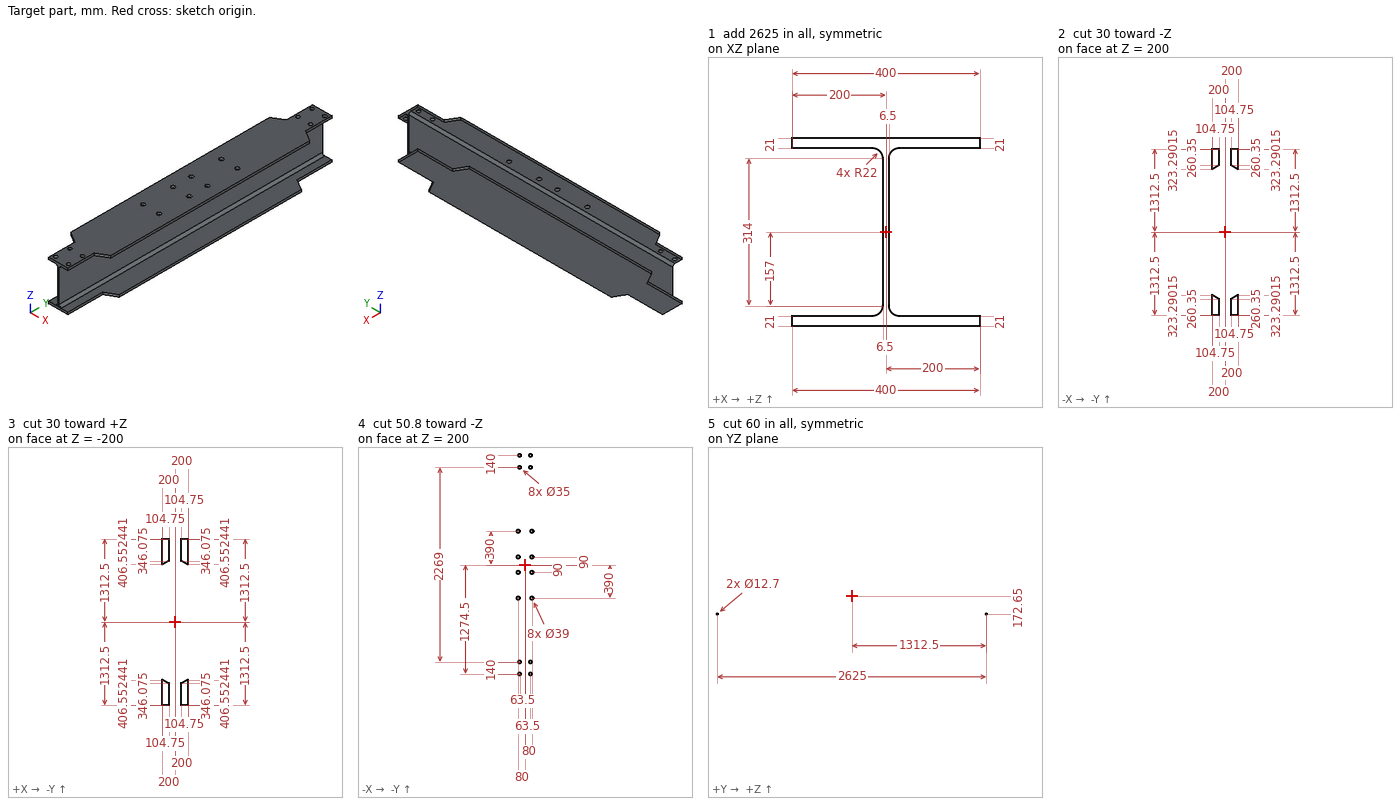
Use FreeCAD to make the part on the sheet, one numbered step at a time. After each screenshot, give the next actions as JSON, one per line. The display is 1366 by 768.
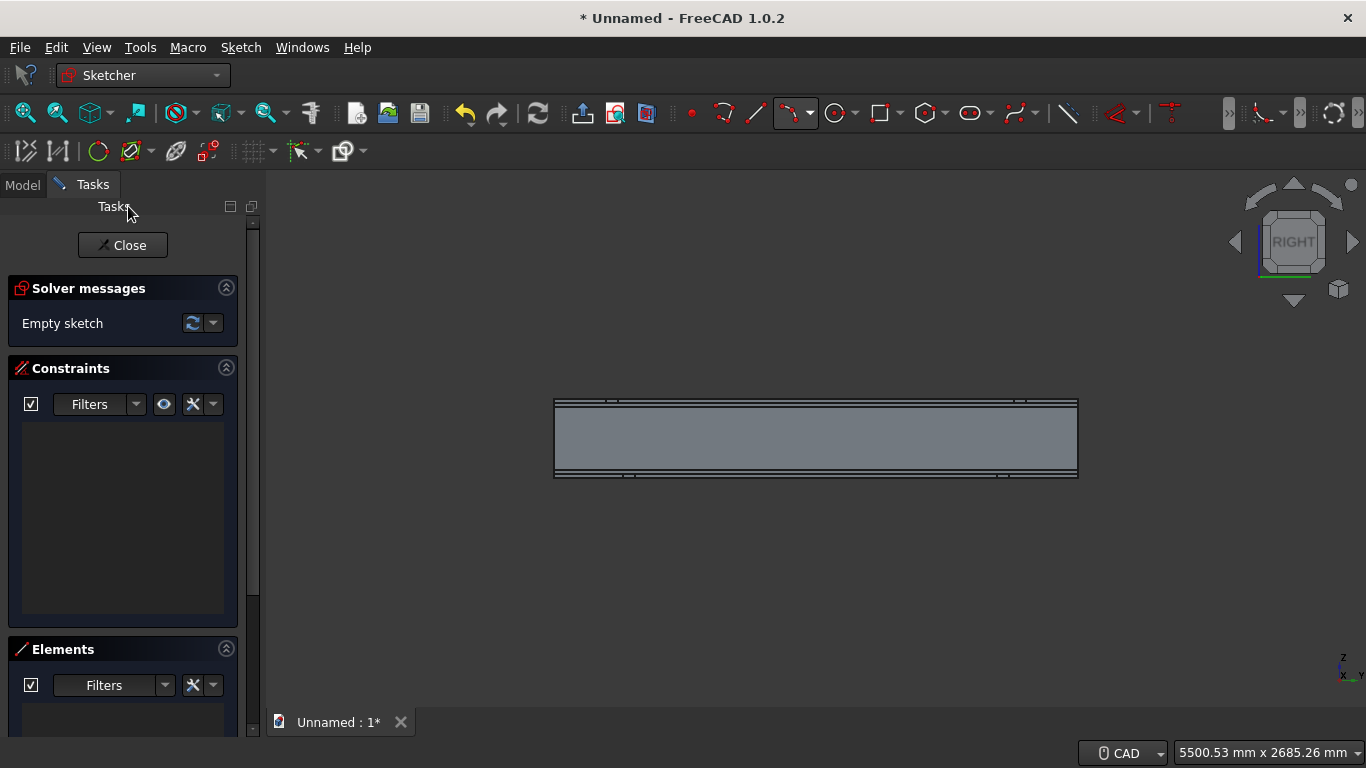
{"action": "left_click", "coordinate": [648, 114]}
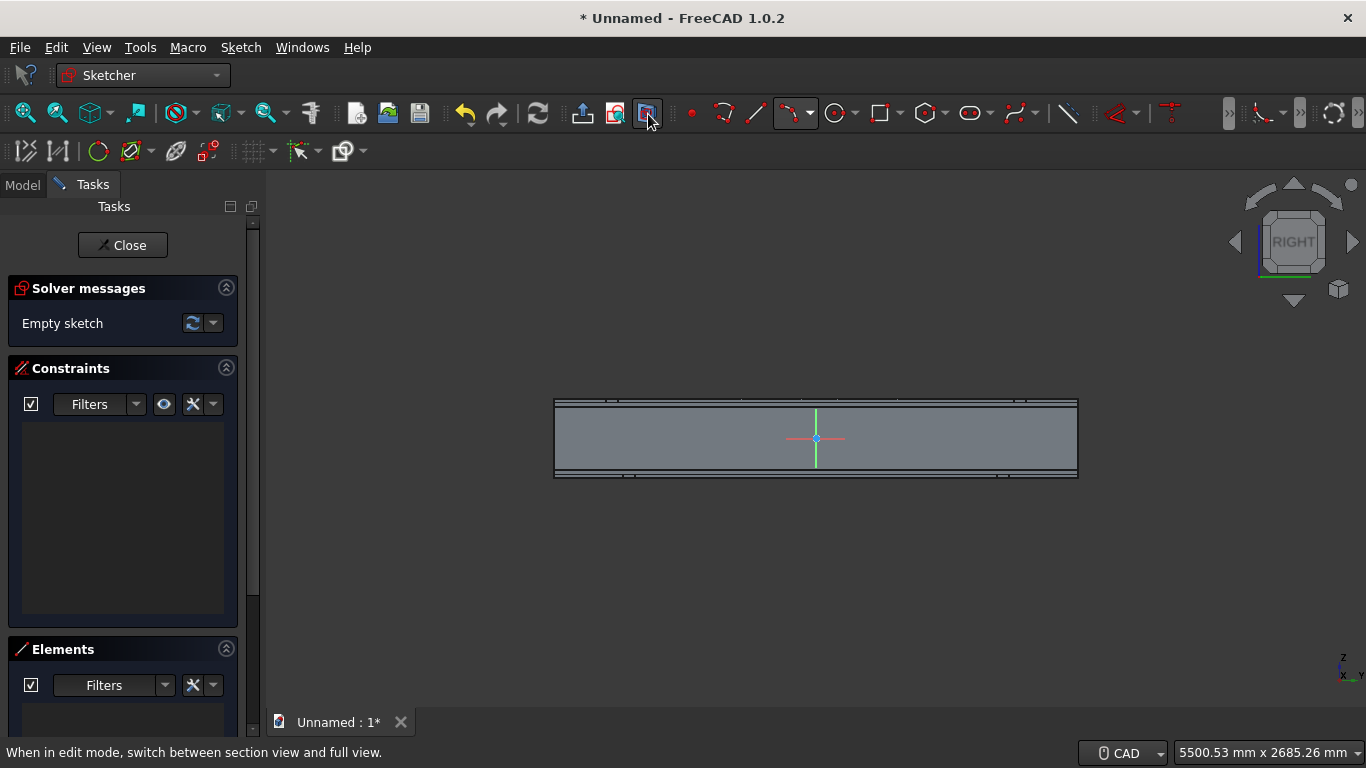
{"action": "left_click", "coordinate": [836, 114]}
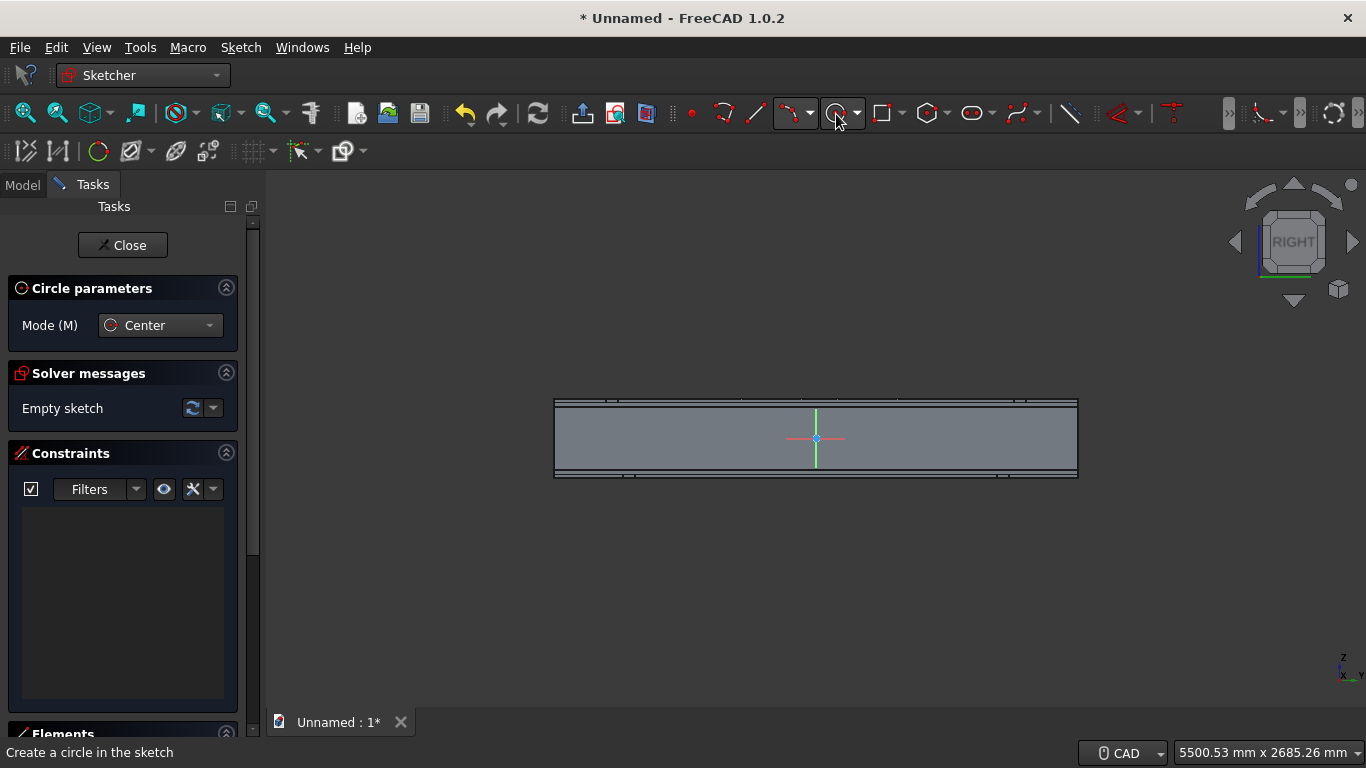
{"action": "scroll", "coordinate": [1078, 473], "scroll_direction": "up", "scroll_amount": 15}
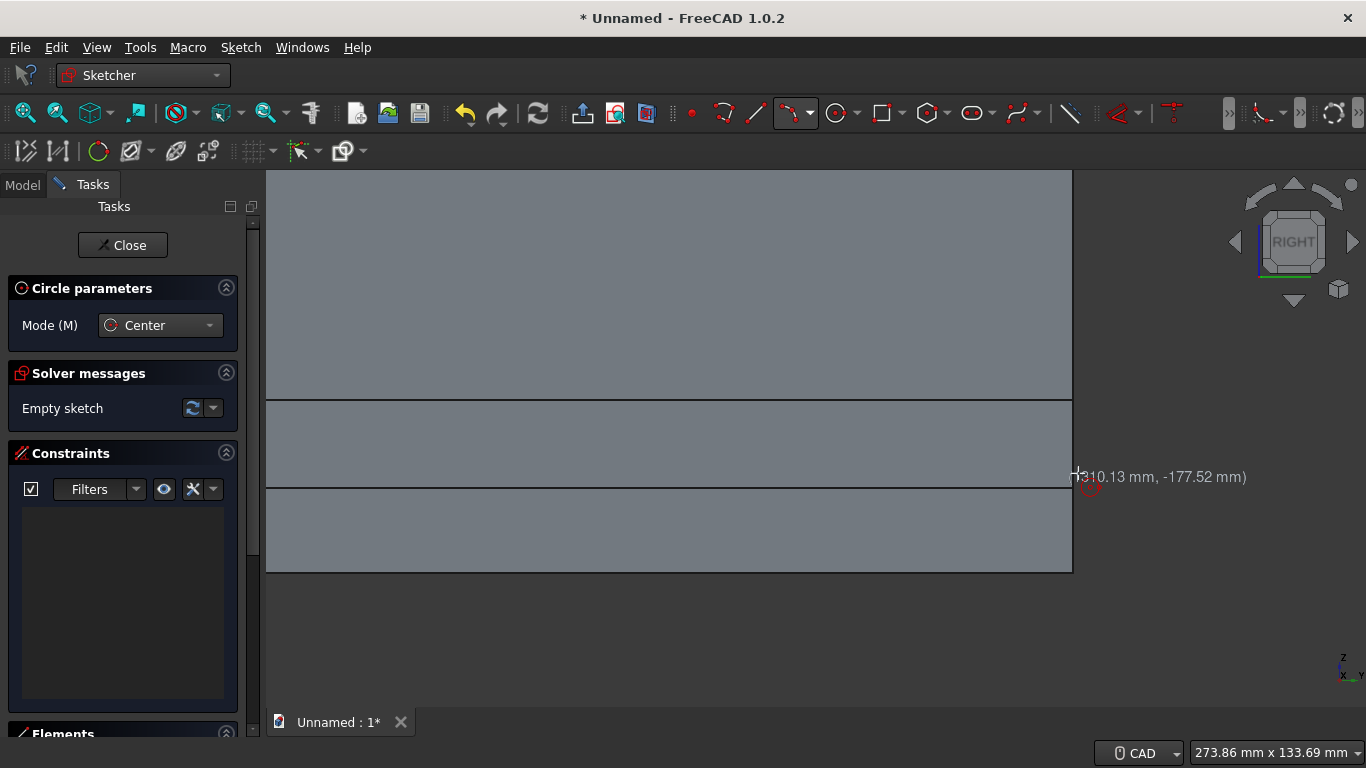
{"action": "scroll", "coordinate": [1068, 459], "scroll_direction": "down", "scroll_amount": 14}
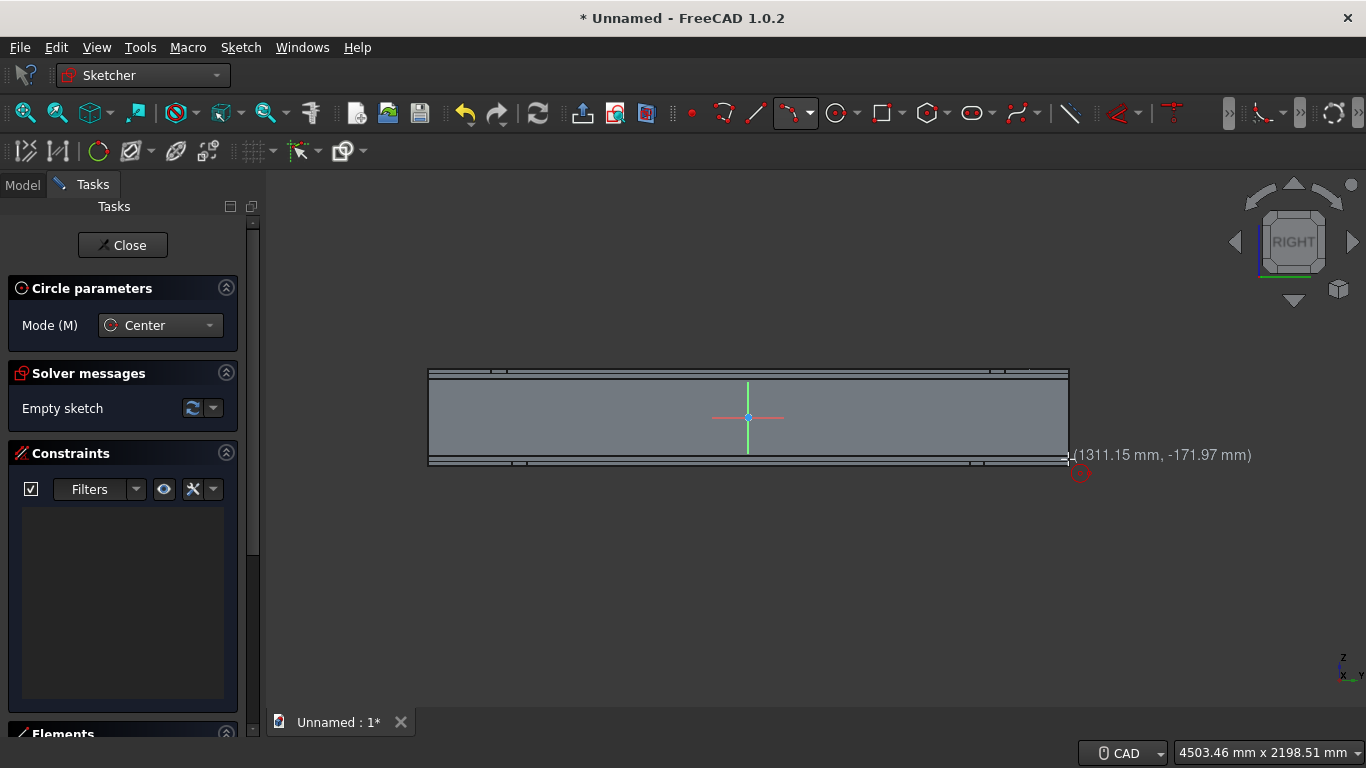
{"action": "left_click", "coordinate": [1069, 460]}
{"action": "mouse_move", "coordinate": [1070, 459]}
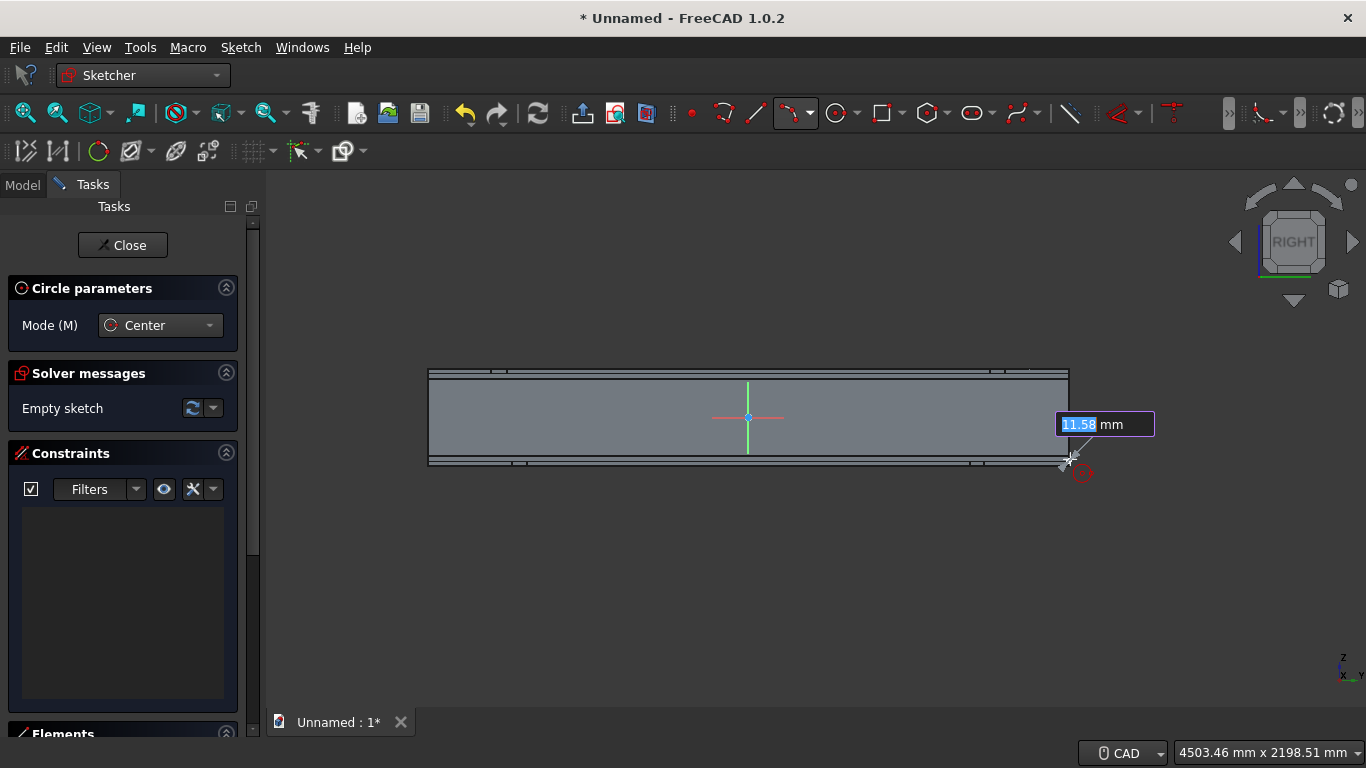
{"action": "type", "text": "12.7"}
{"action": "key", "text": "Return"}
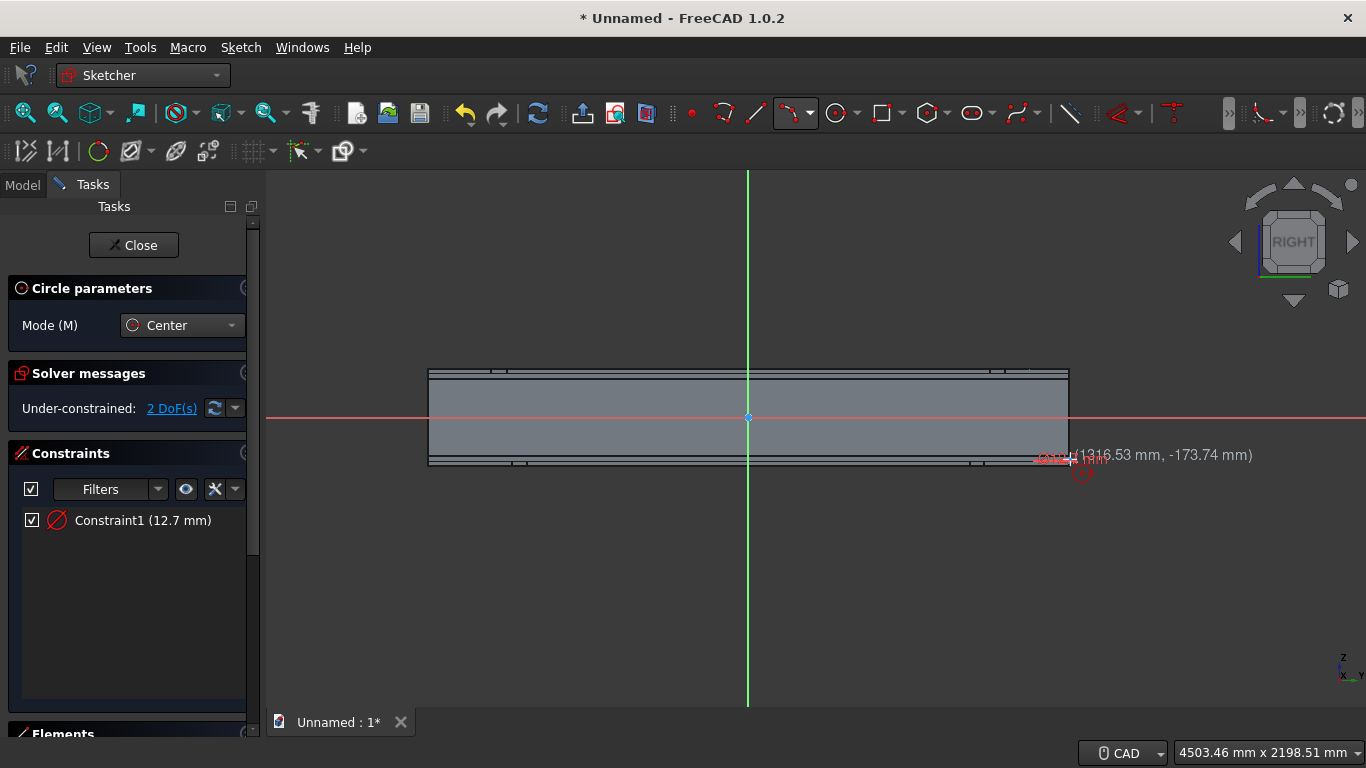
{"action": "scroll", "coordinate": [428, 460], "scroll_direction": "up", "scroll_amount": 14}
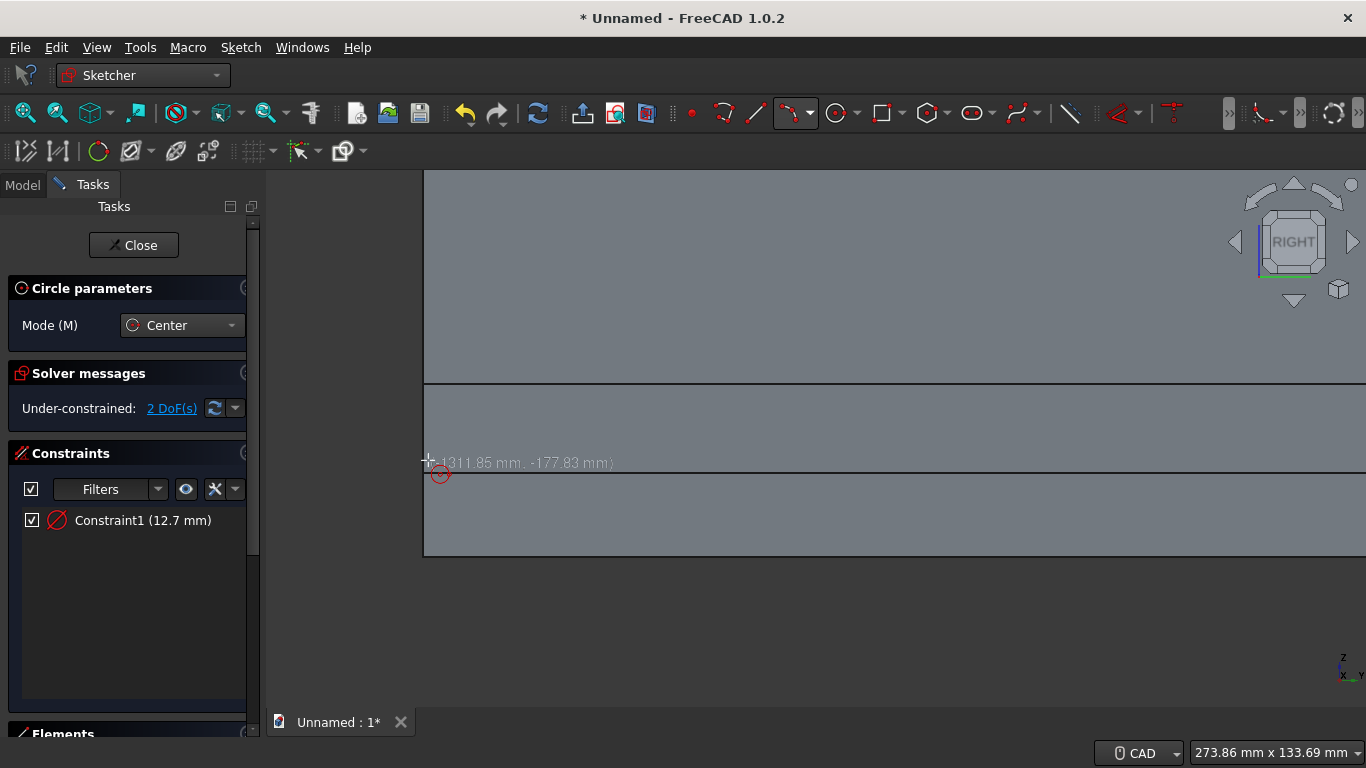
{"action": "scroll", "coordinate": [427, 460], "scroll_direction": "down", "scroll_amount": 14}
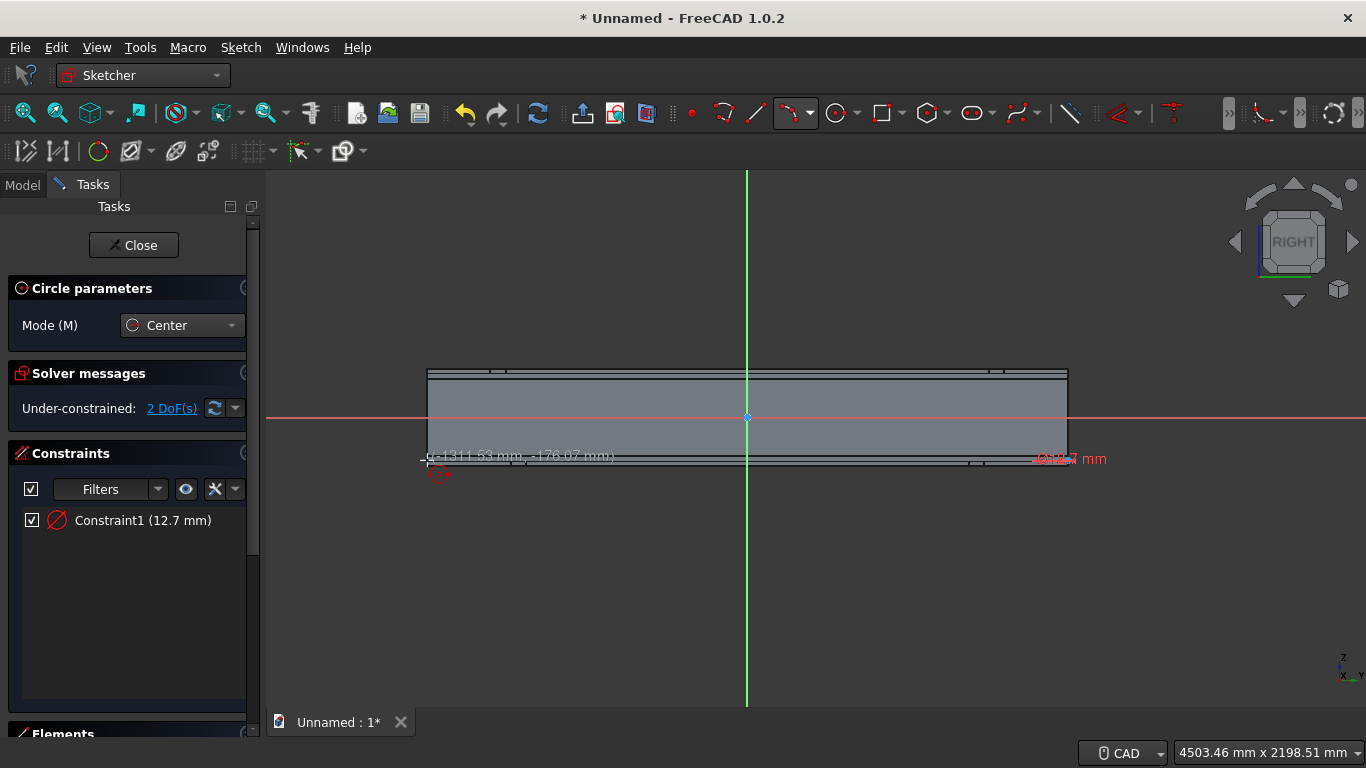
{"action": "left_click", "coordinate": [427, 460]}
{"action": "mouse_move", "coordinate": [428, 459]}